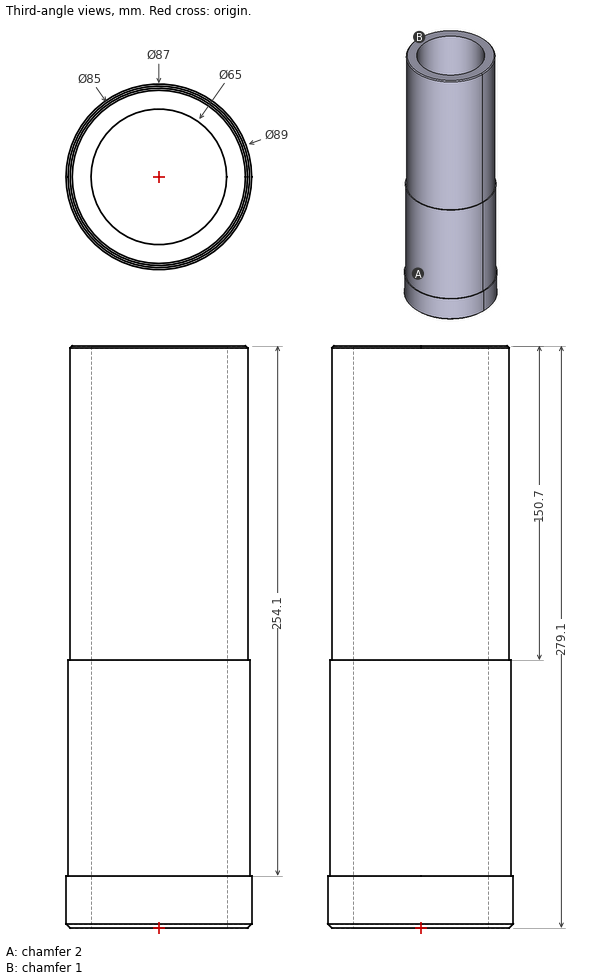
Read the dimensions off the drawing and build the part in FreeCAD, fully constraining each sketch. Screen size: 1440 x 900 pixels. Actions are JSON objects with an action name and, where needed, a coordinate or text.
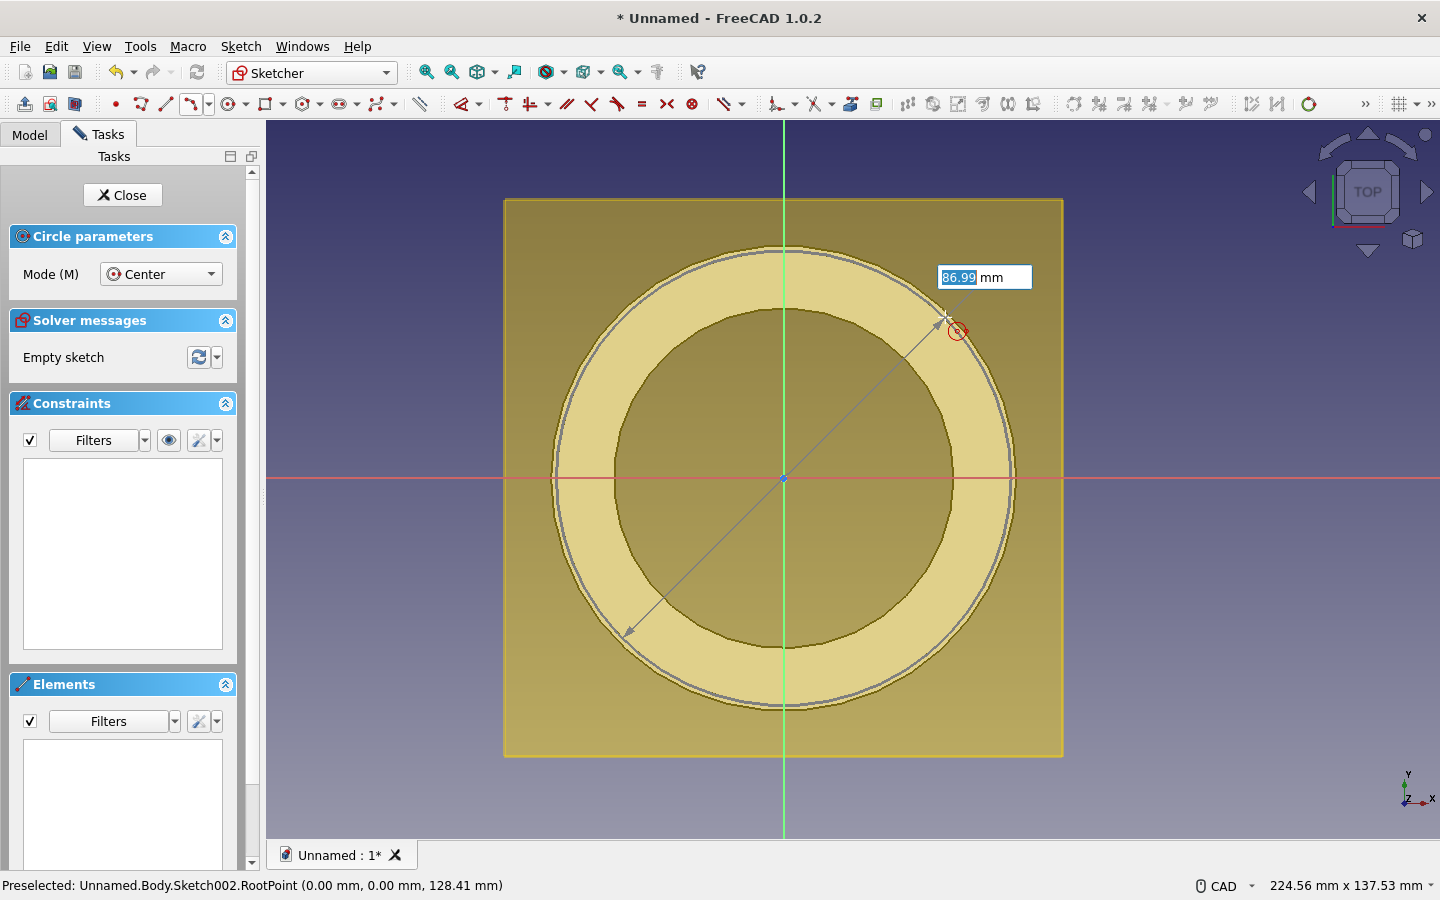
{"action": "type", "text": "87"}
{"action": "key", "text": "Return"}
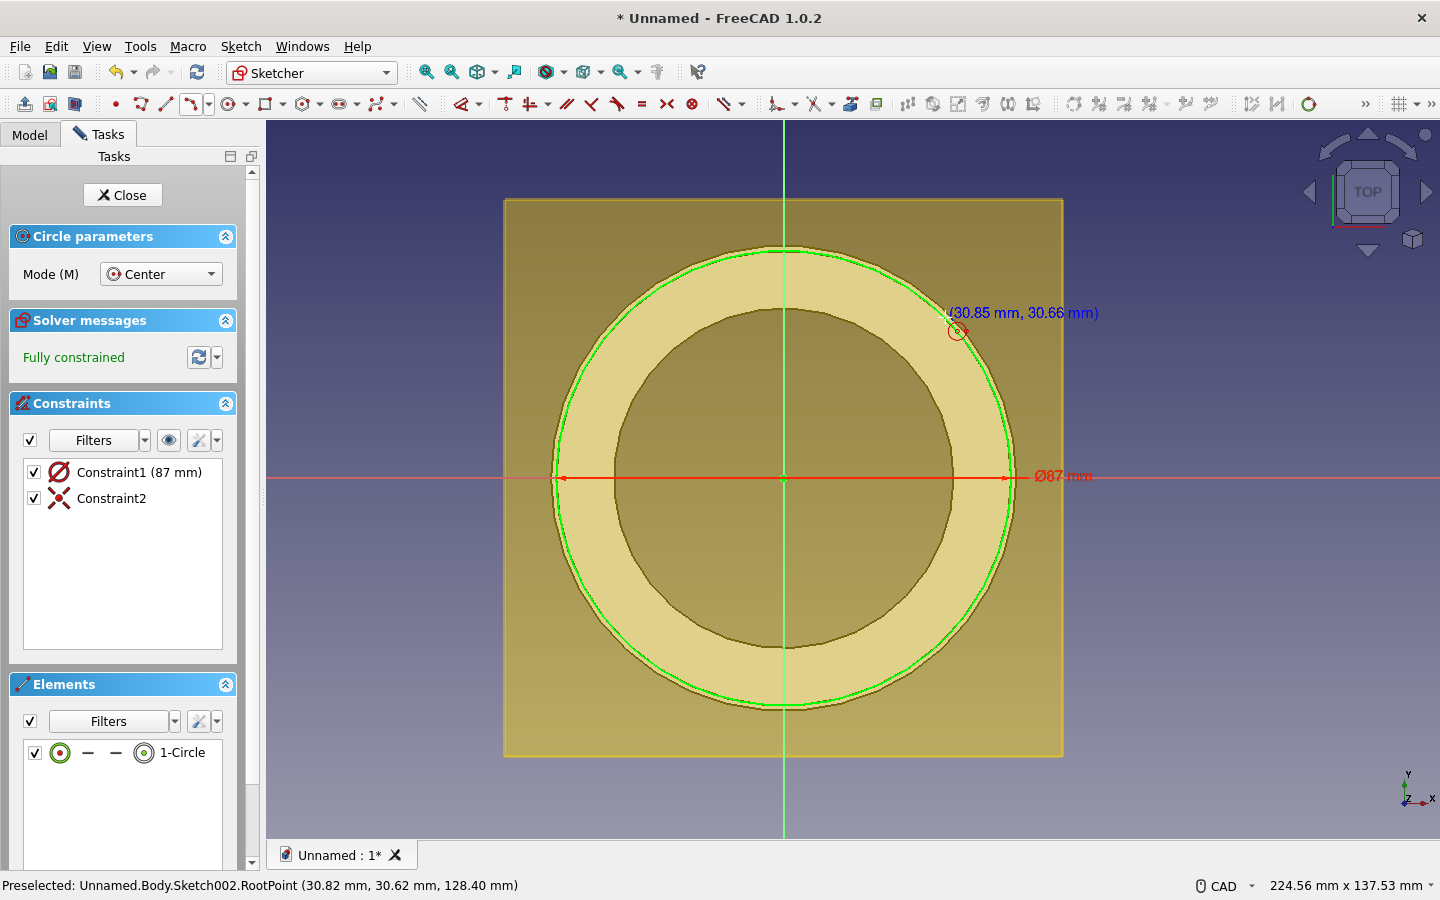
{"action": "left_click", "coordinate": [784, 478]}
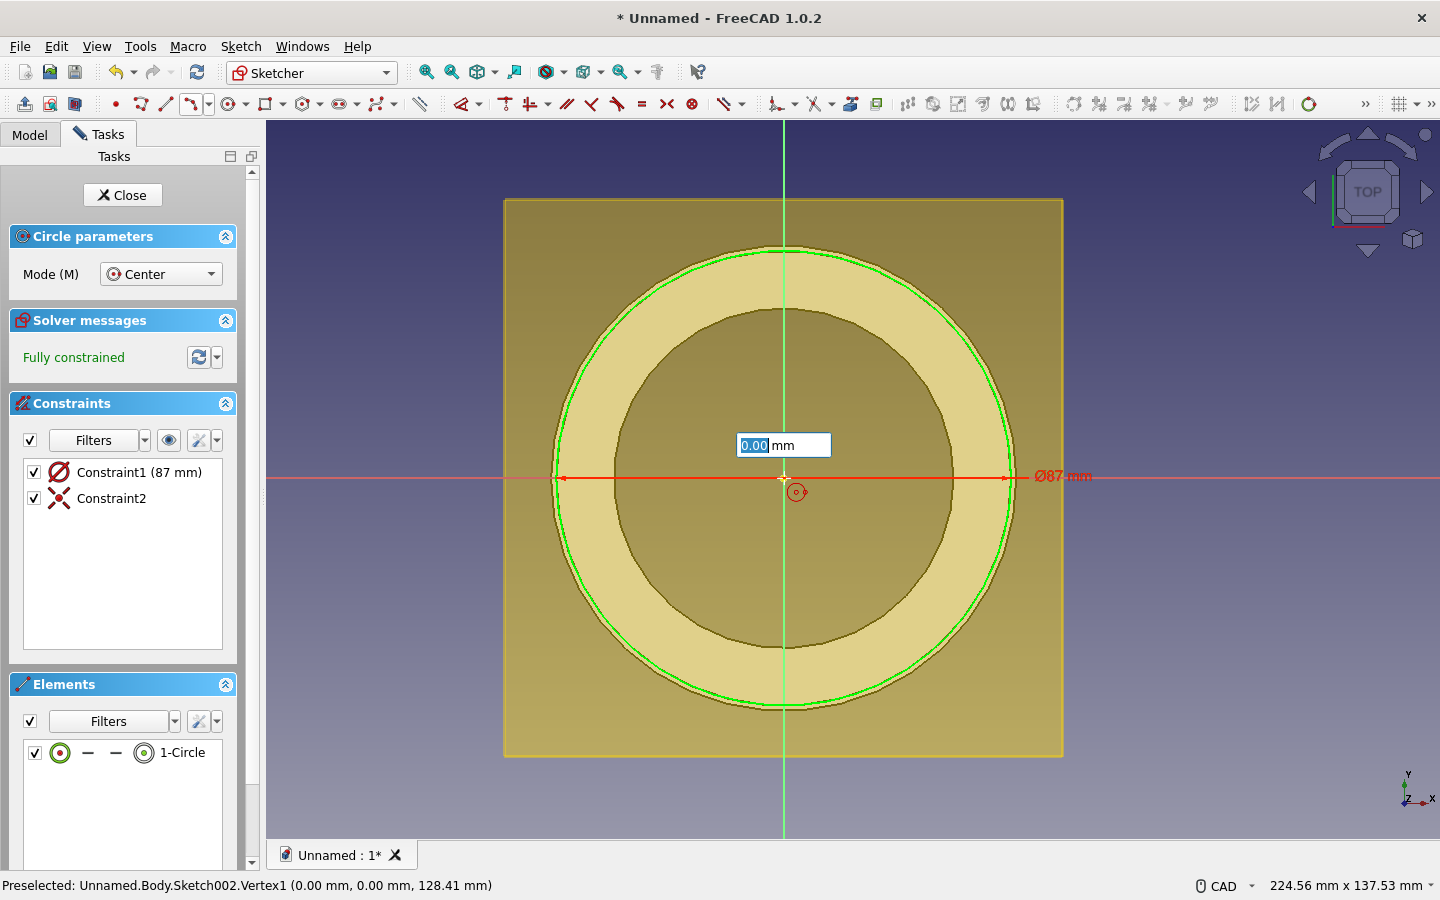
{"action": "scroll", "coordinate": [941, 321], "scroll_direction": "up", "scroll_amount": 6}
{"action": "mouse_move", "coordinate": [939, 321]}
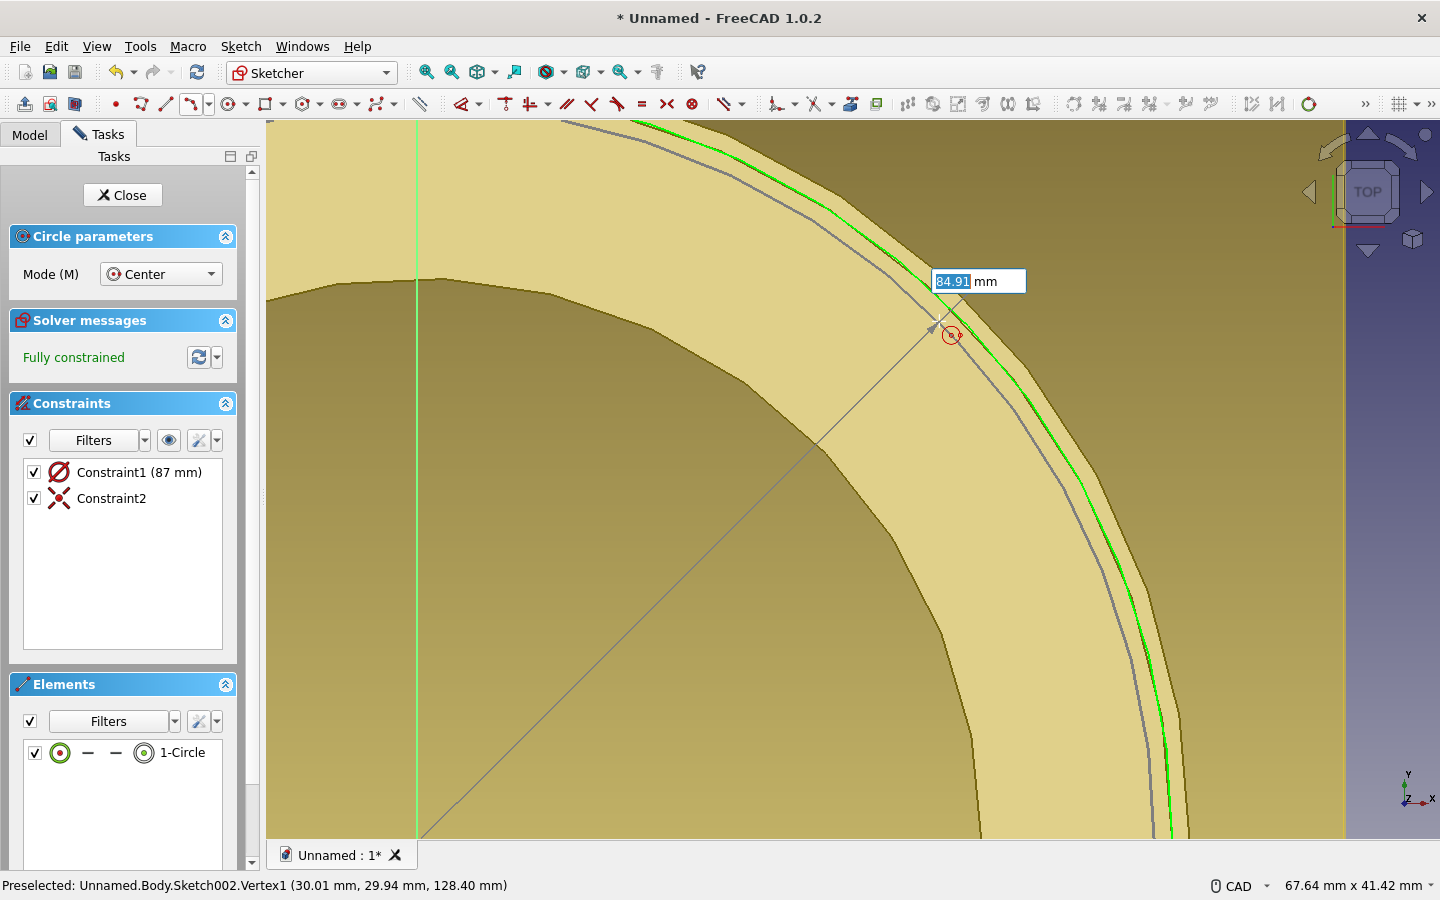
{"action": "type", "text": "85"}
{"action": "key", "text": "Return"}
{"action": "key", "text": "Escape"}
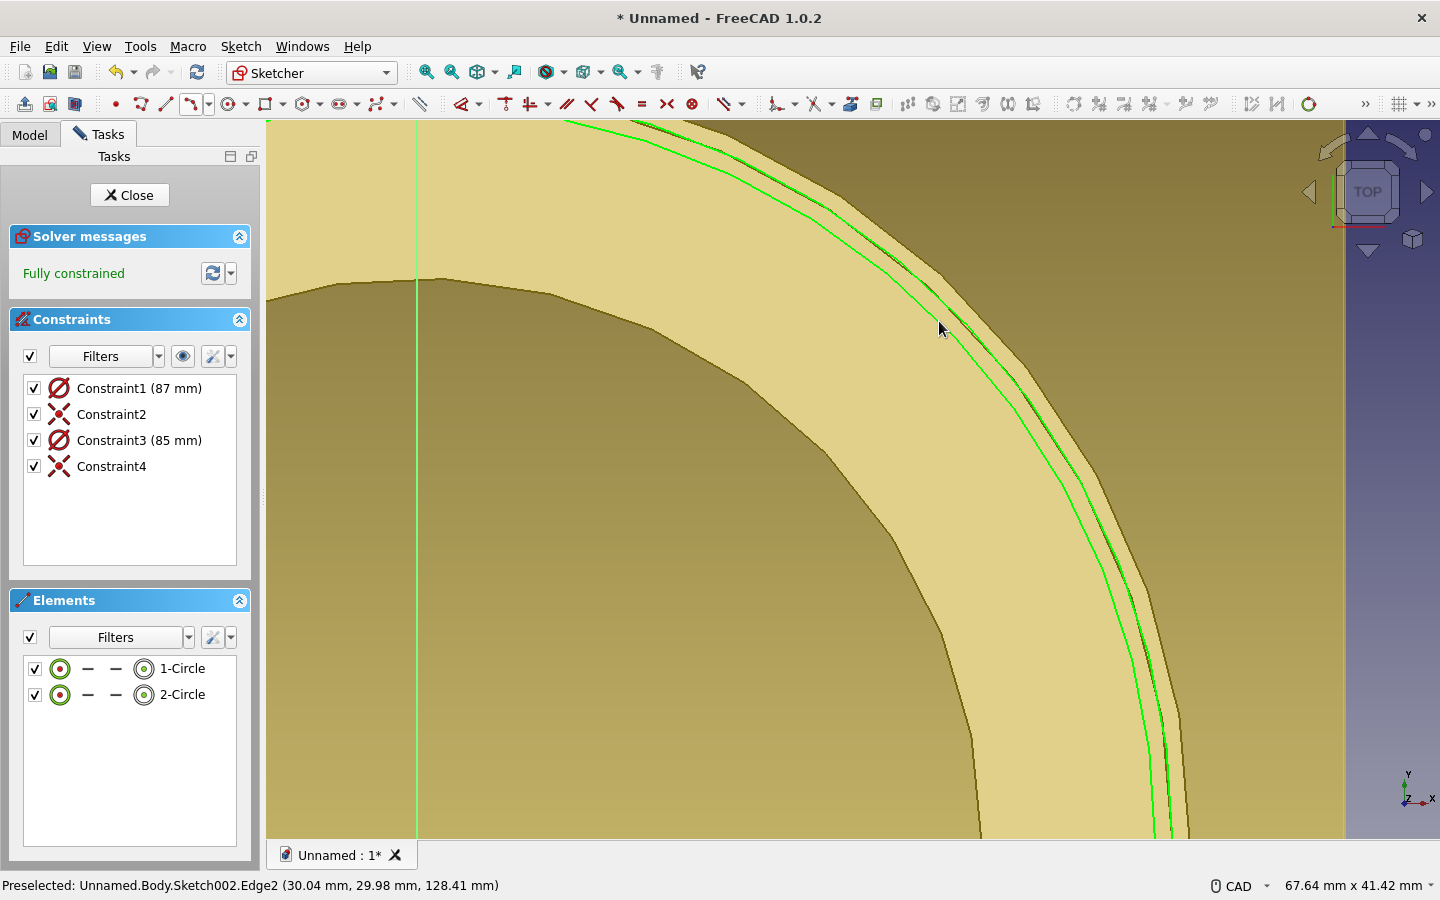
{"action": "left_click", "coordinate": [130, 195]}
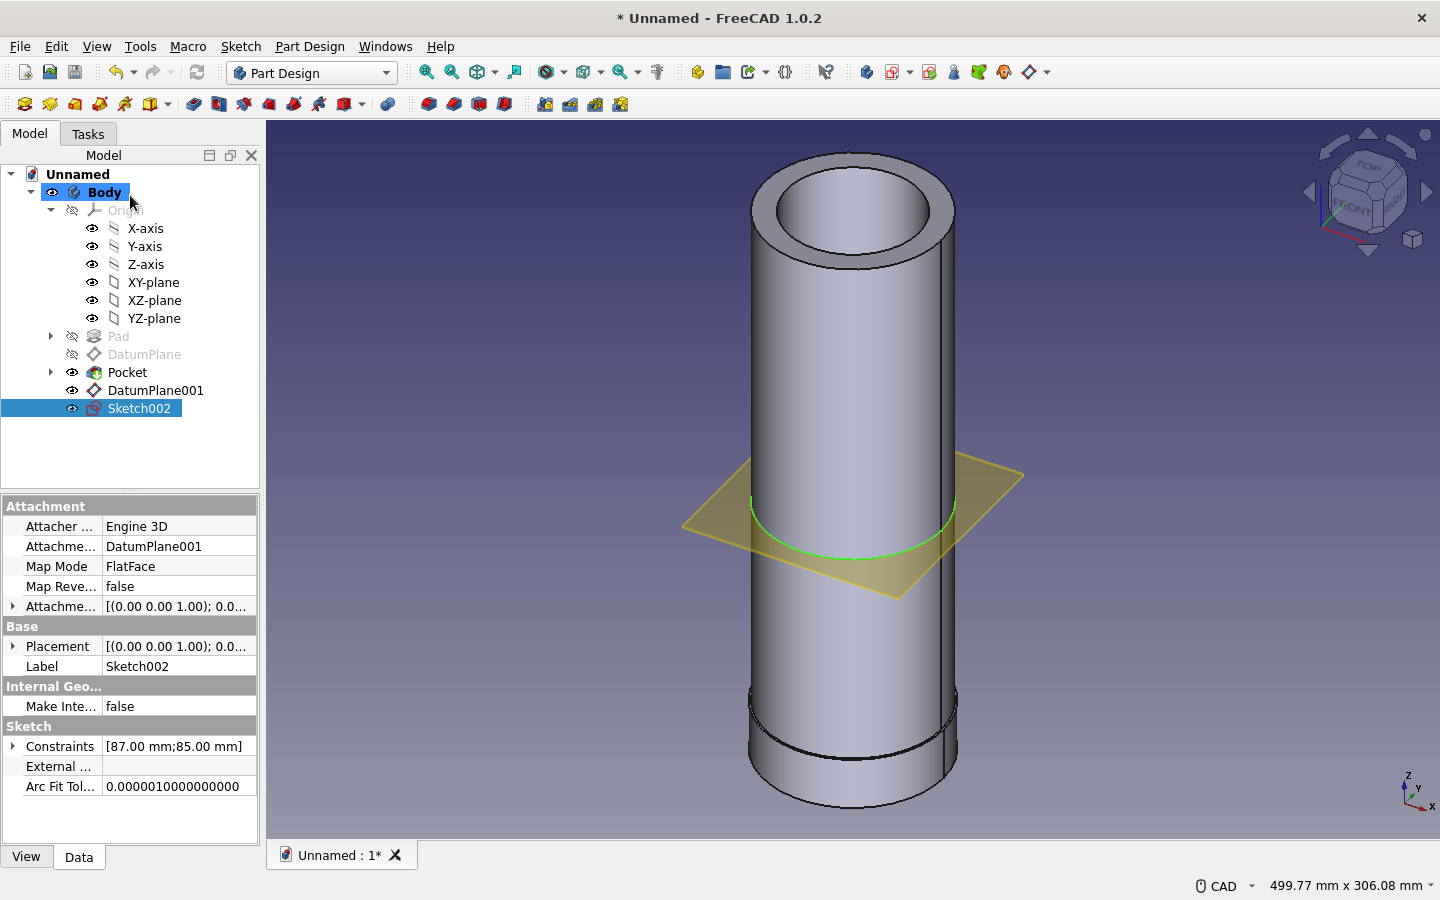
{"action": "left_click", "coordinate": [194, 104]}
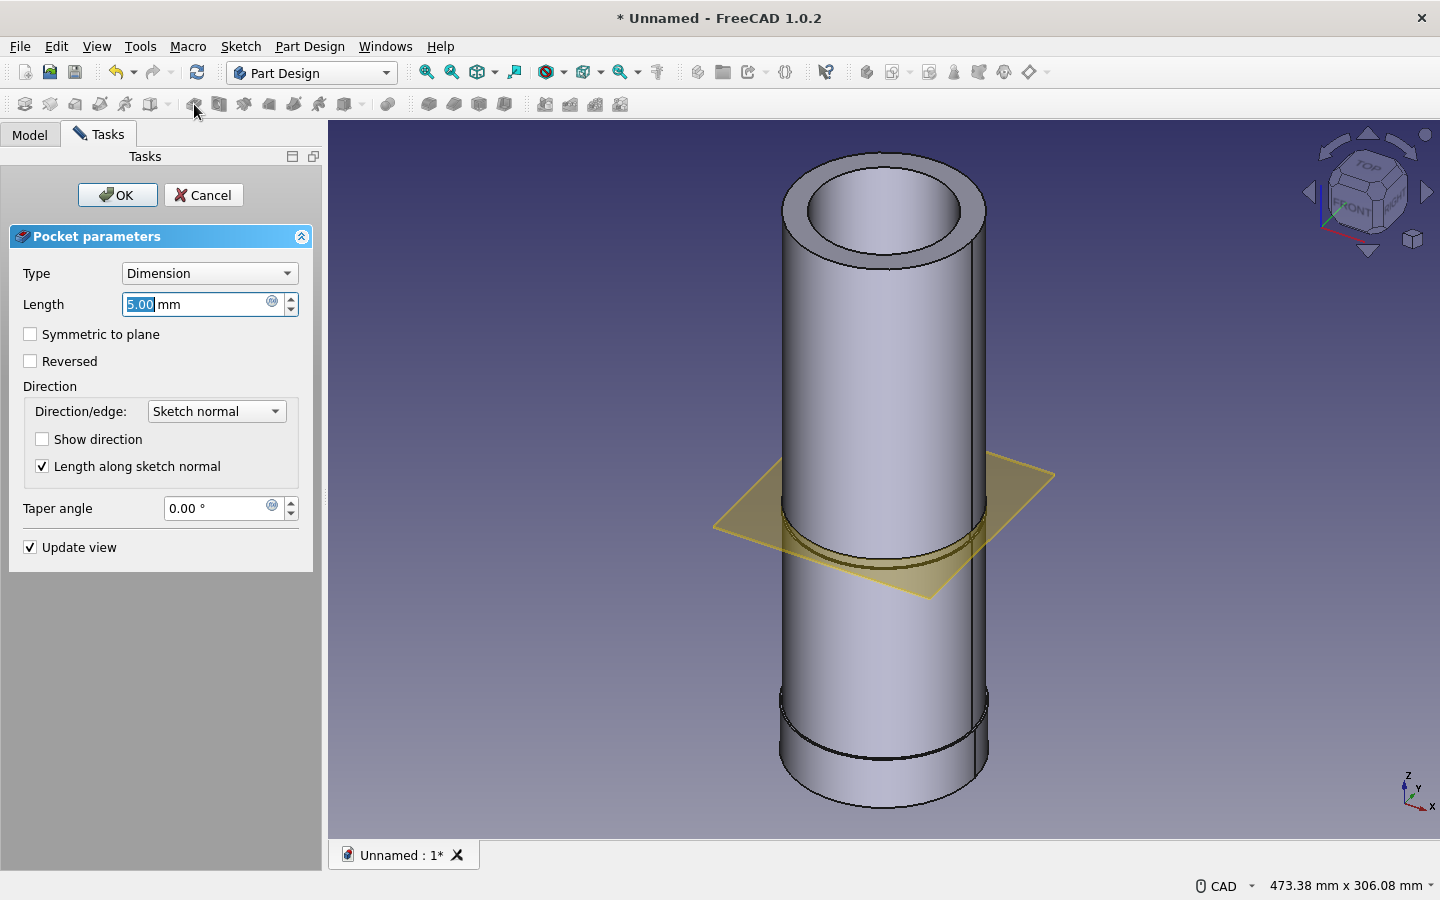
{"action": "type", "text": "150.7"}
{"action": "key", "text": "Tab"}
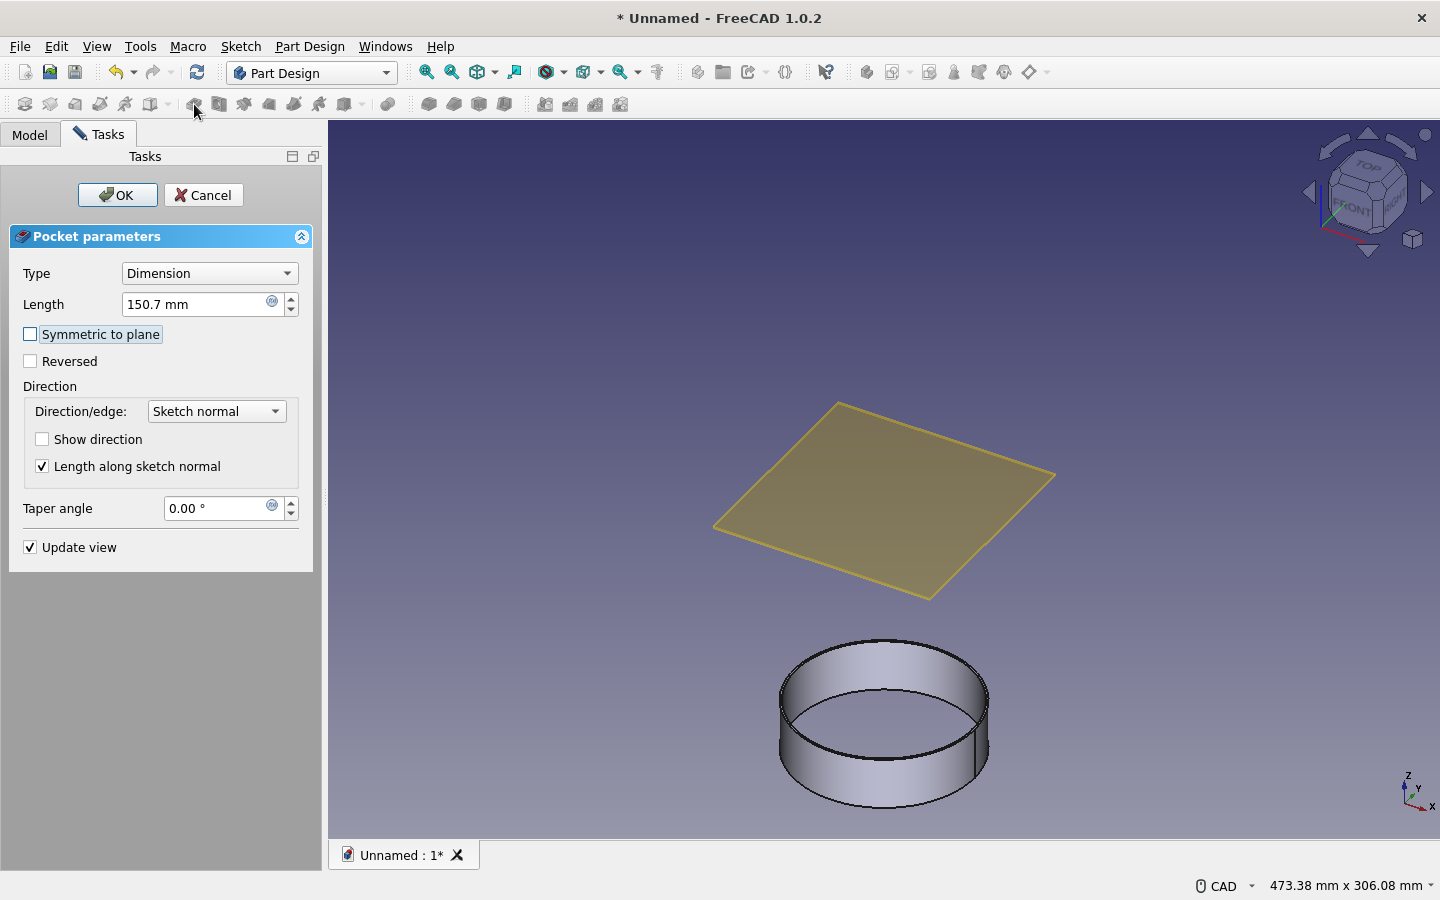
{"action": "left_click", "coordinate": [31, 361]}